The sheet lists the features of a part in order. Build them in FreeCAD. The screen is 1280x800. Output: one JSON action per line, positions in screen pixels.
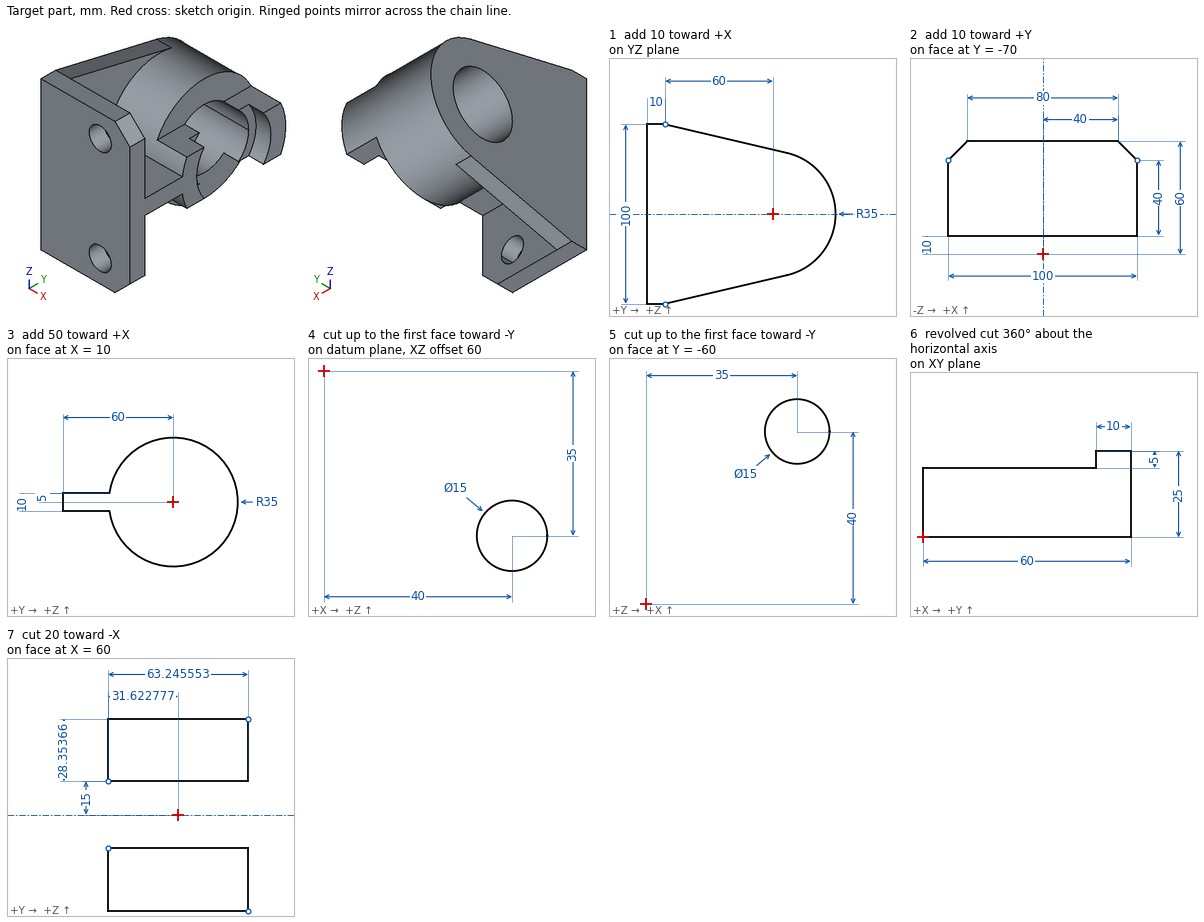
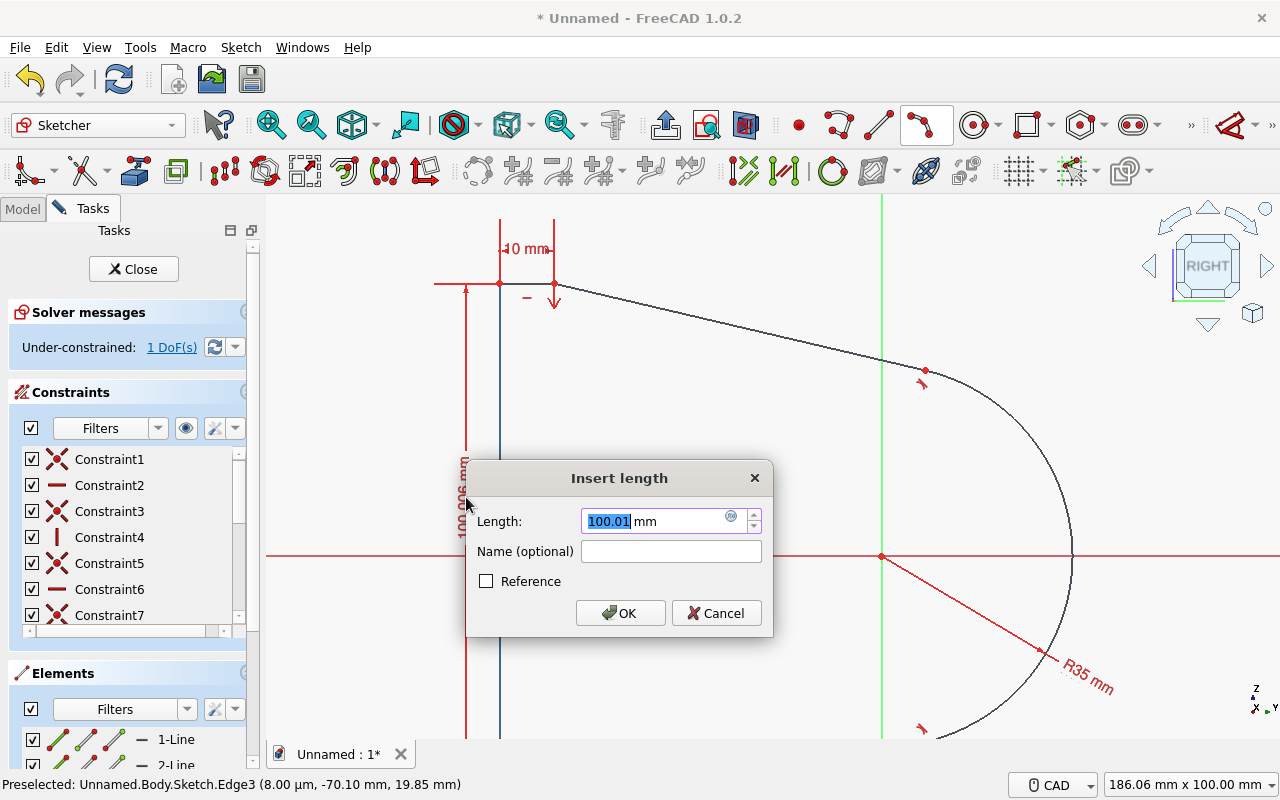
{"action": "type", "text": "100"}
{"action": "key", "text": "Return"}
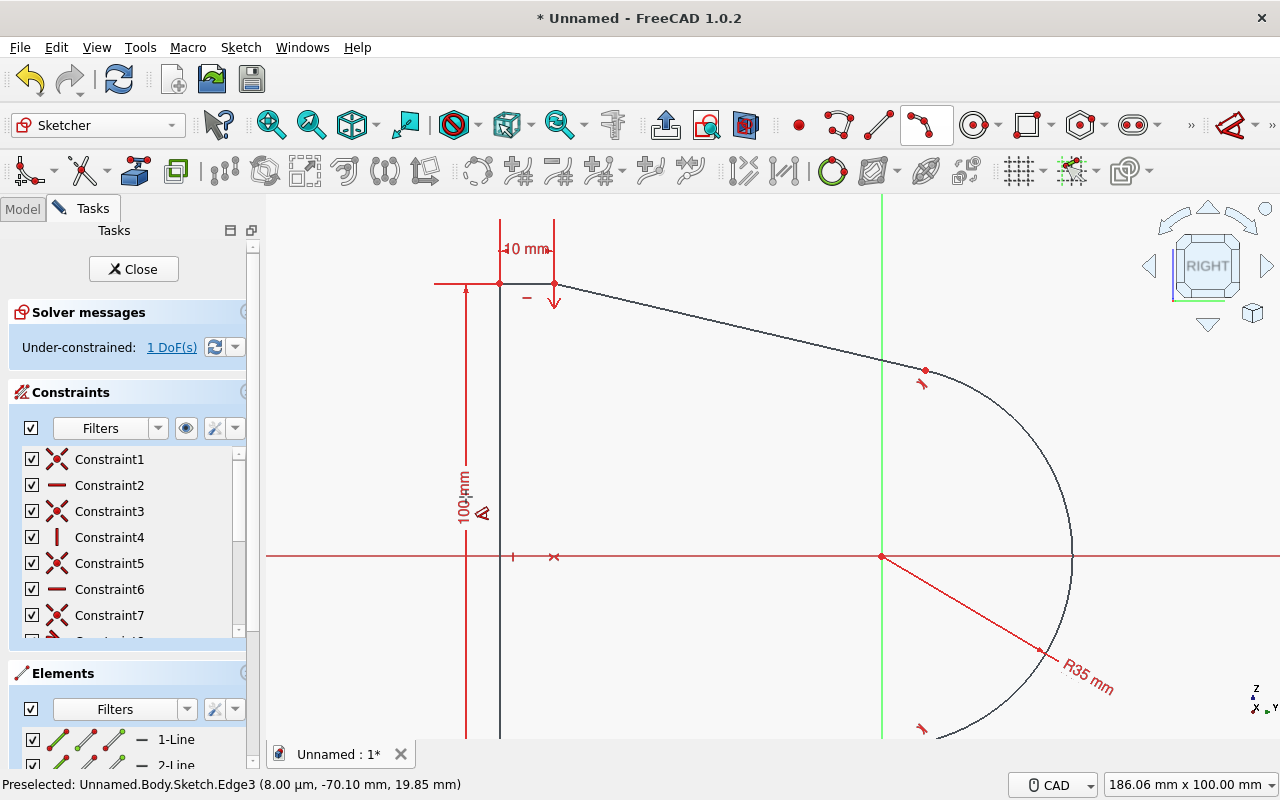
{"action": "left_click", "coordinate": [554, 284]}
{"action": "left_click", "coordinate": [718, 250]}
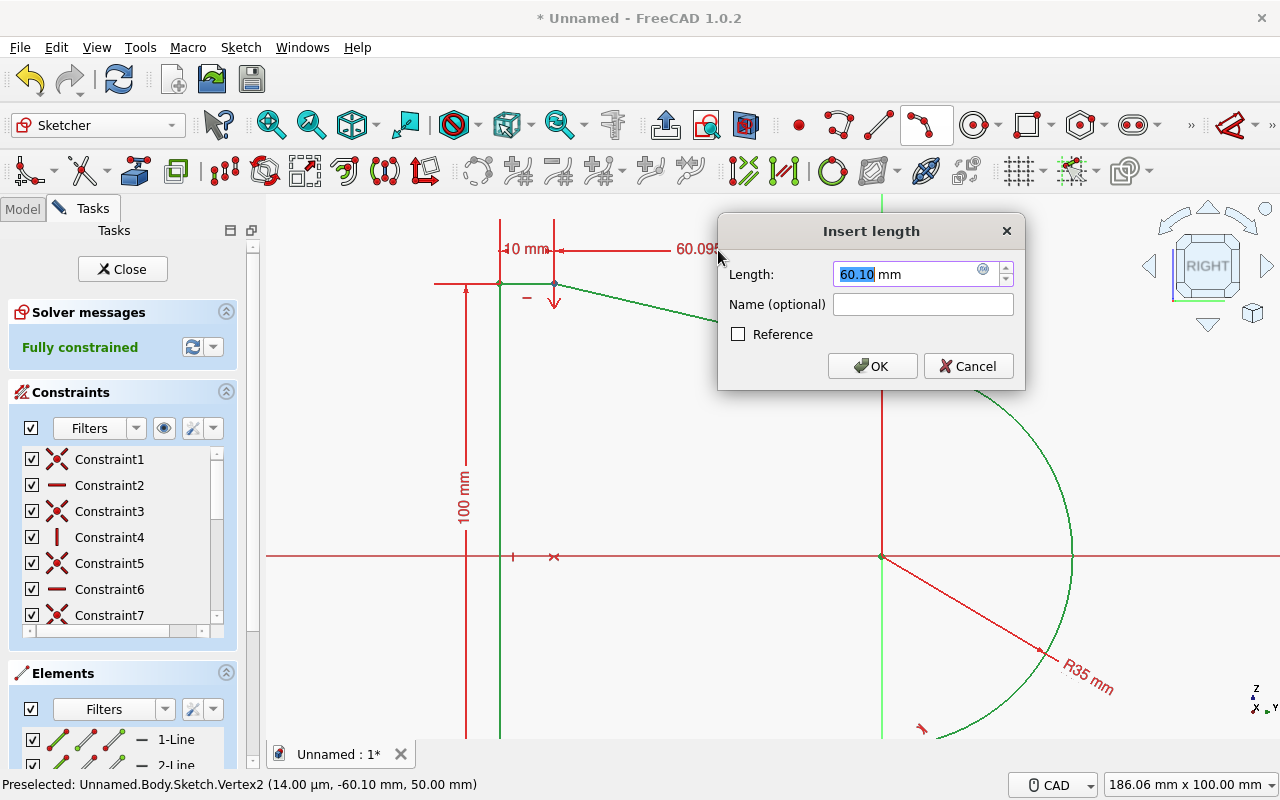
{"action": "type", "text": "60"}
{"action": "key", "text": "Return"}
{"action": "key", "text": "Escape"}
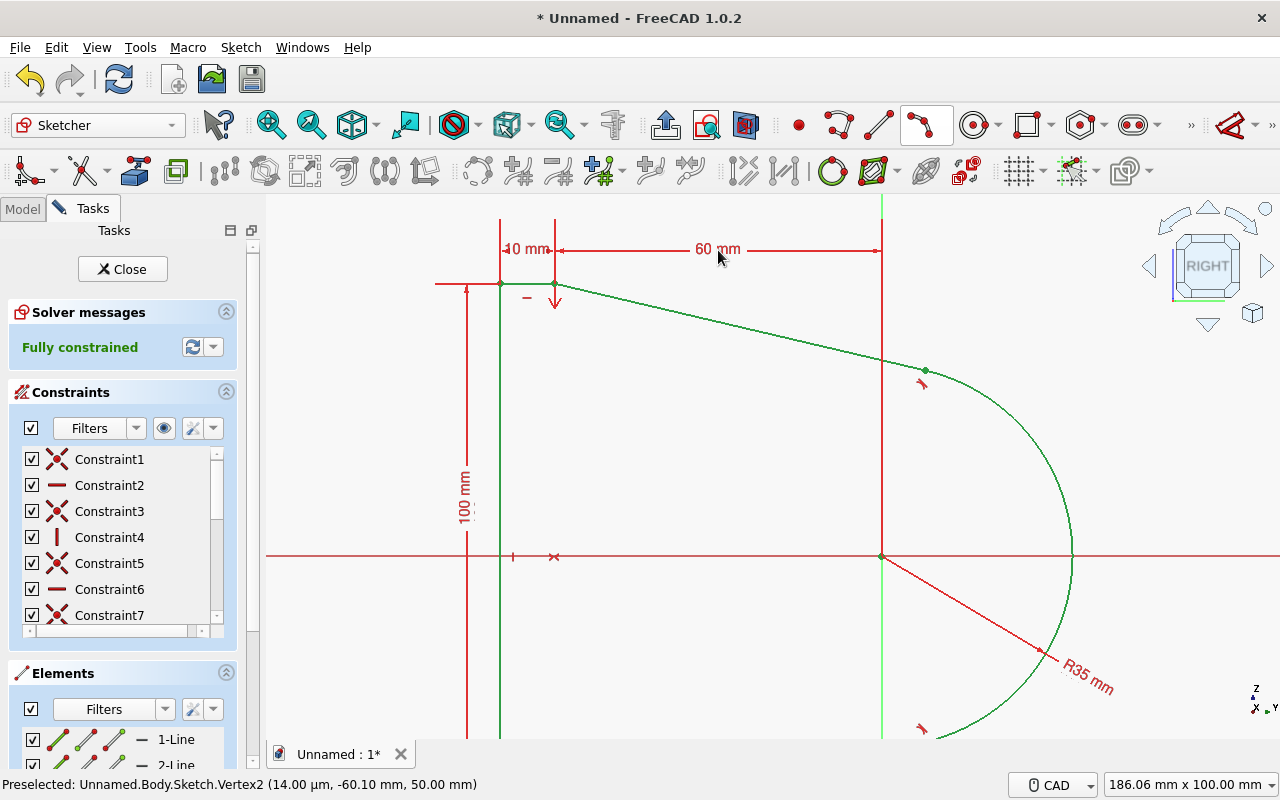
{"action": "left_click", "coordinate": [123, 269]}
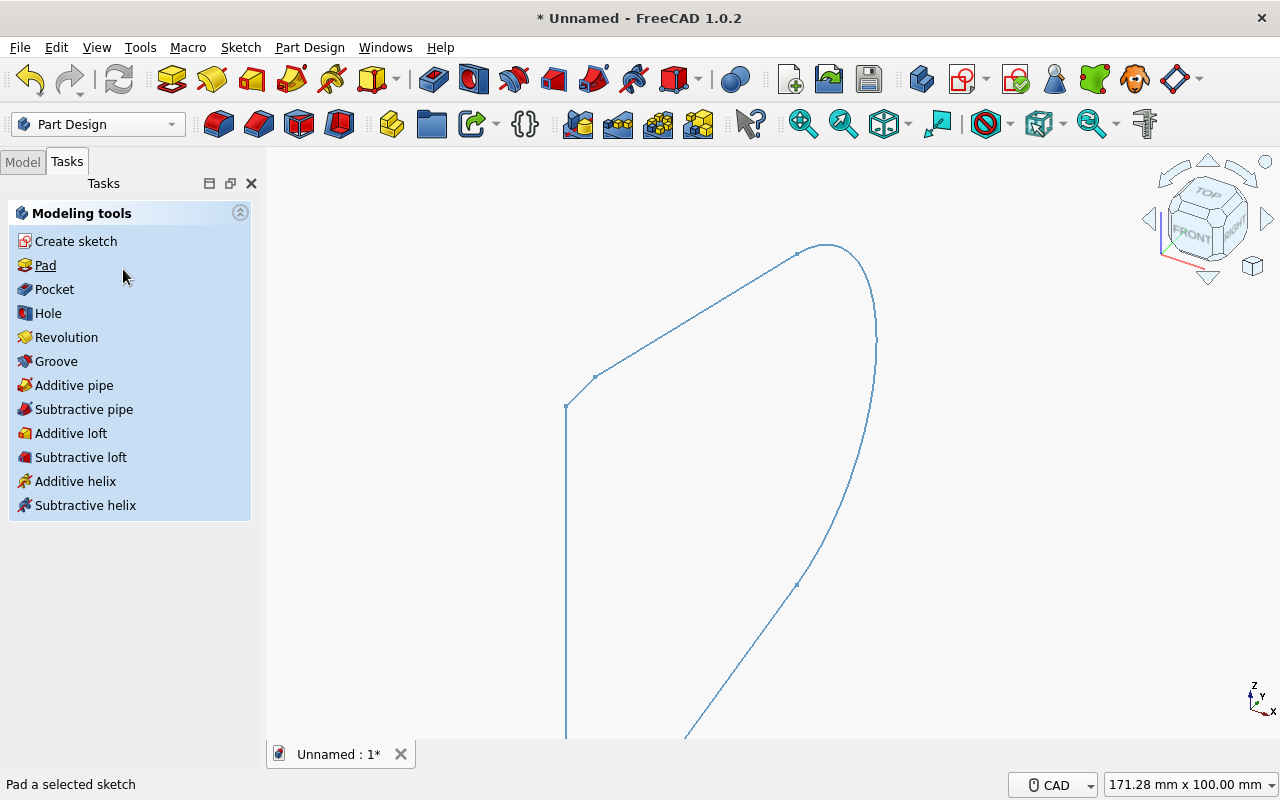
{"action": "left_click", "coordinate": [172, 80]}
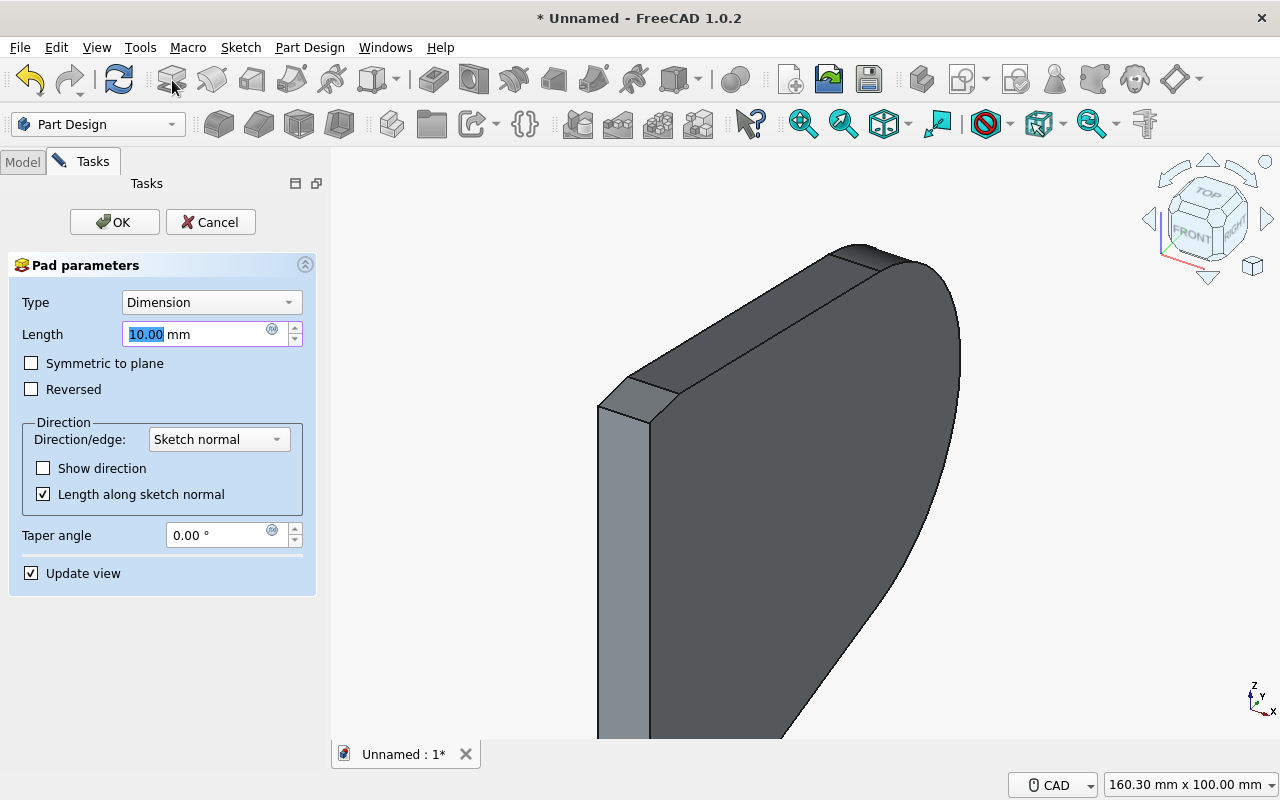
{"action": "type", "text": "10"}
{"action": "key", "text": "Tab"}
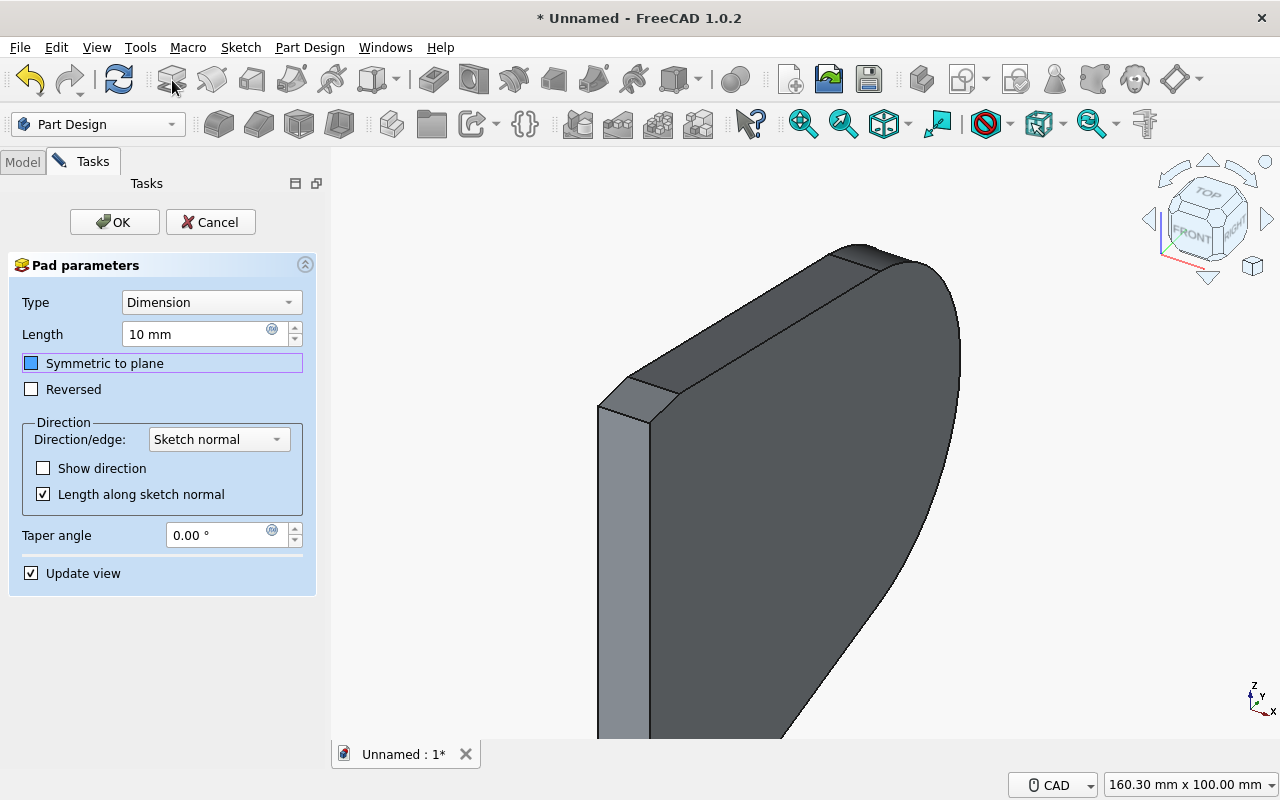
{"action": "left_click", "coordinate": [115, 222]}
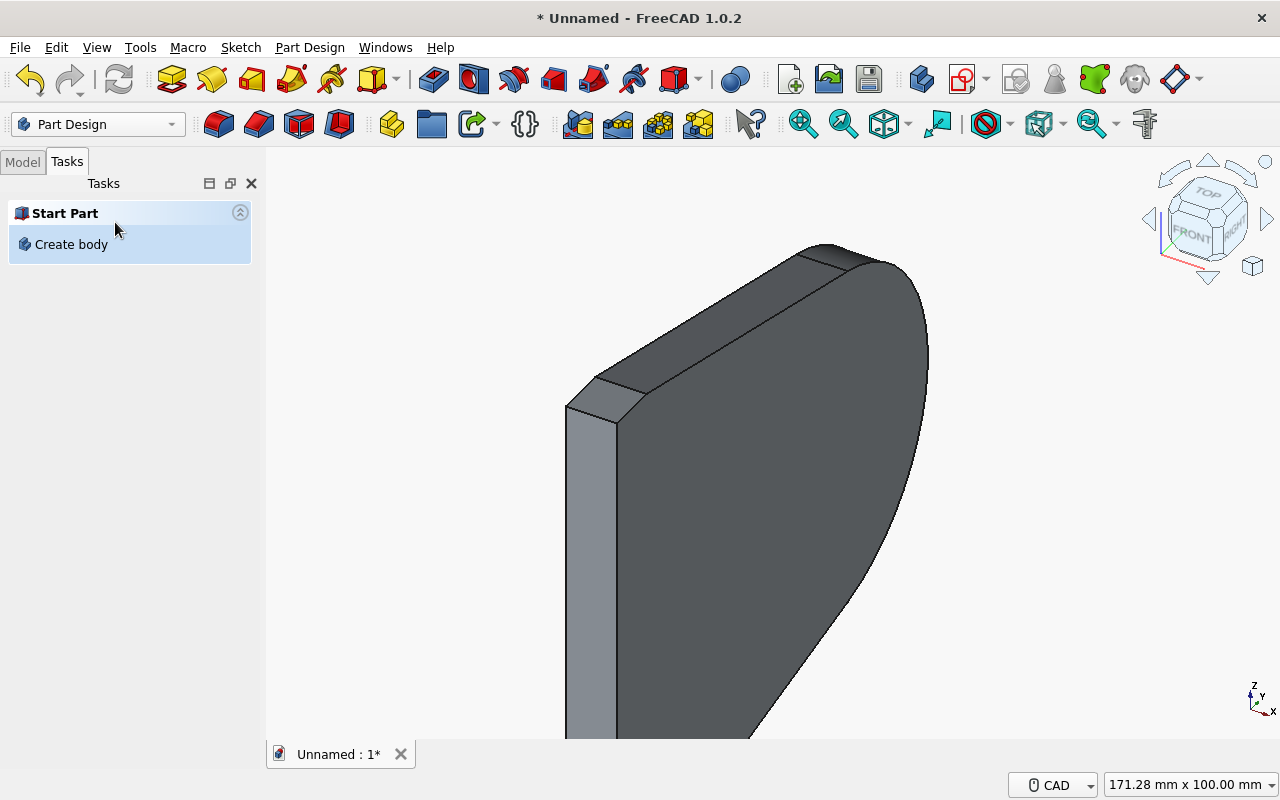
{"action": "left_click", "coordinate": [804, 124]}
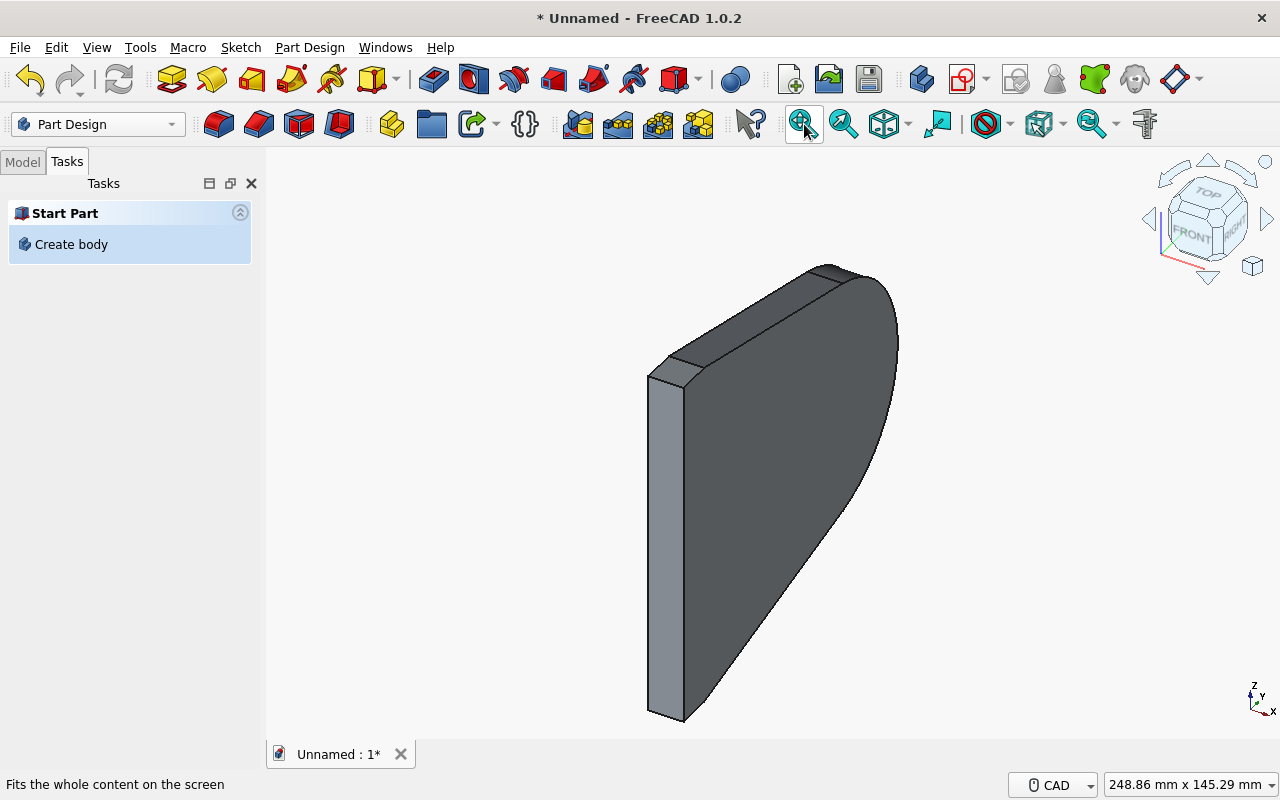
{"action": "left_click", "coordinate": [666, 644]}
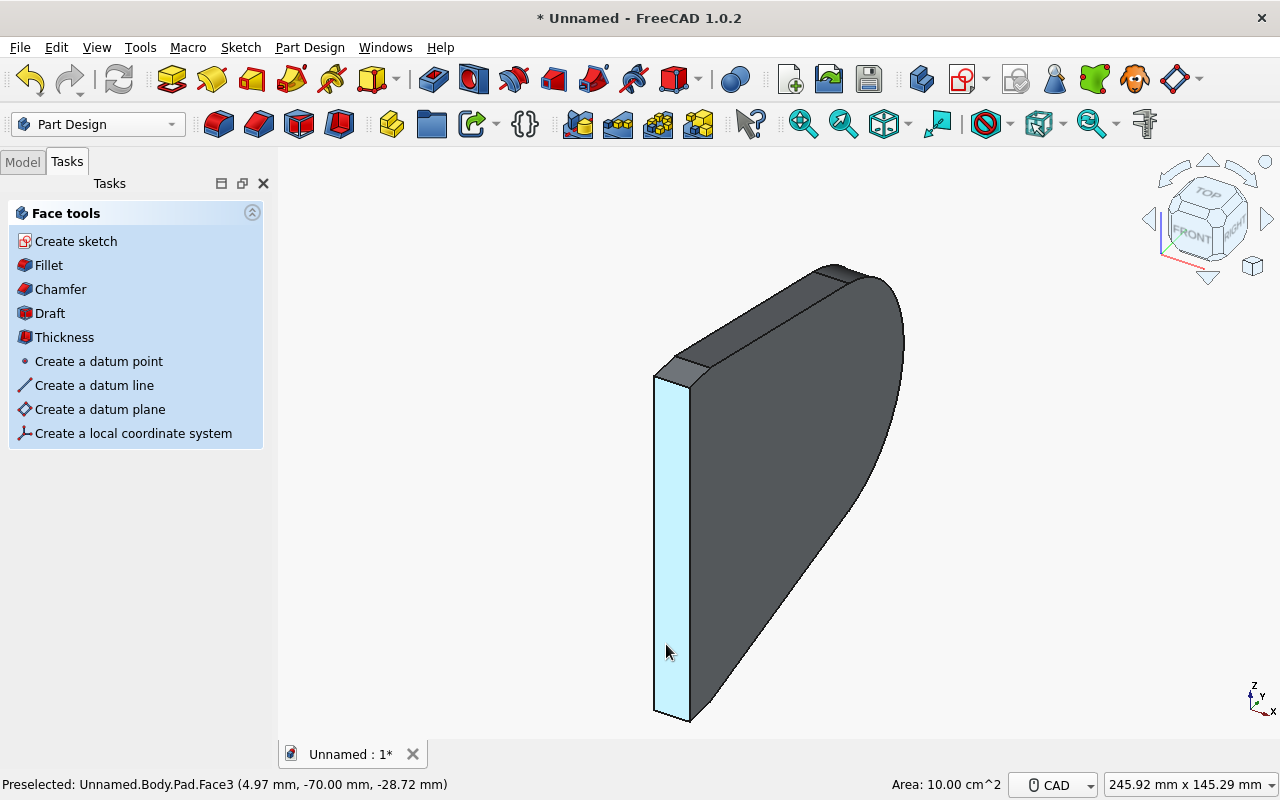
{"action": "left_click", "coordinate": [962, 80]}